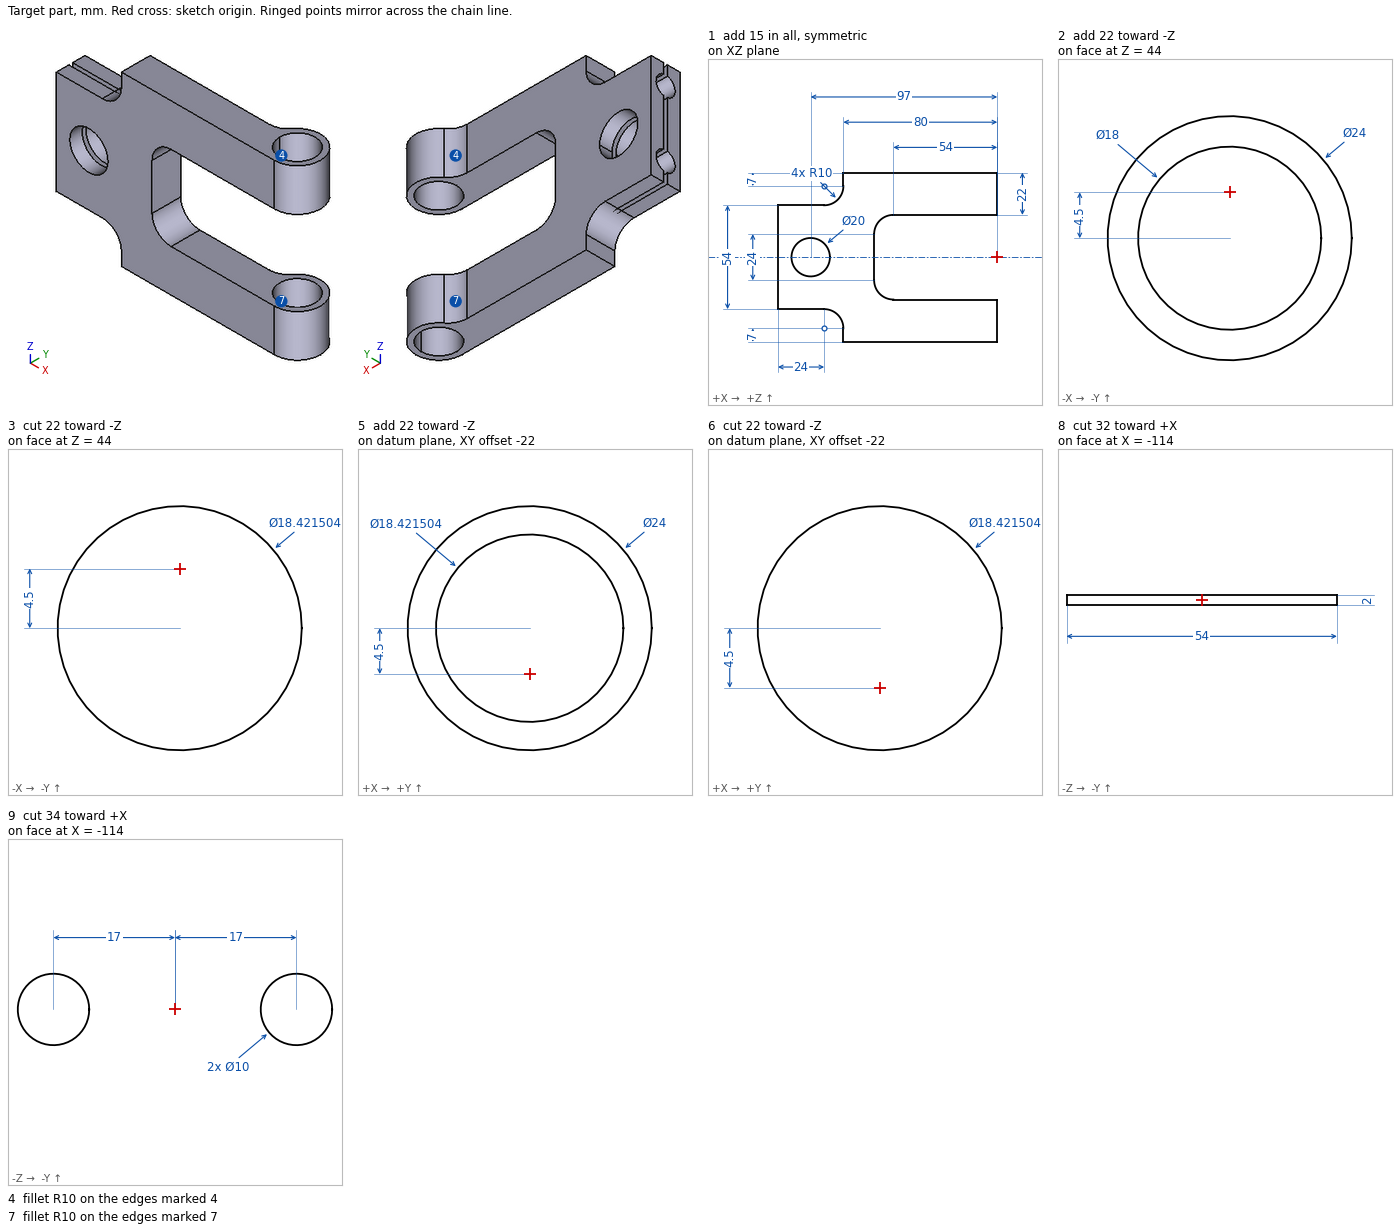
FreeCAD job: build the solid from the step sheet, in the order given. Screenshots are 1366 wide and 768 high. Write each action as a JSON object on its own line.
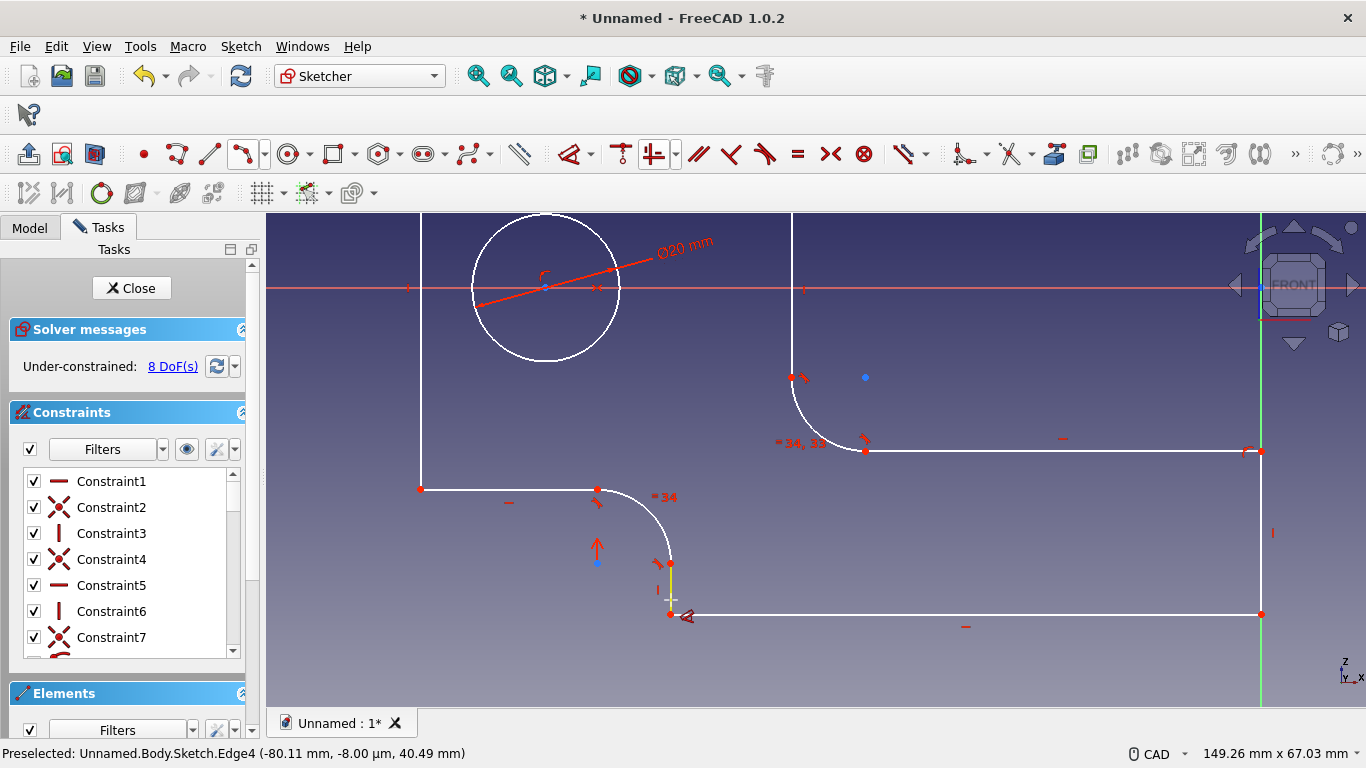
{"action": "left_click", "coordinate": [671, 599]}
{"action": "left_click", "coordinate": [637, 589]}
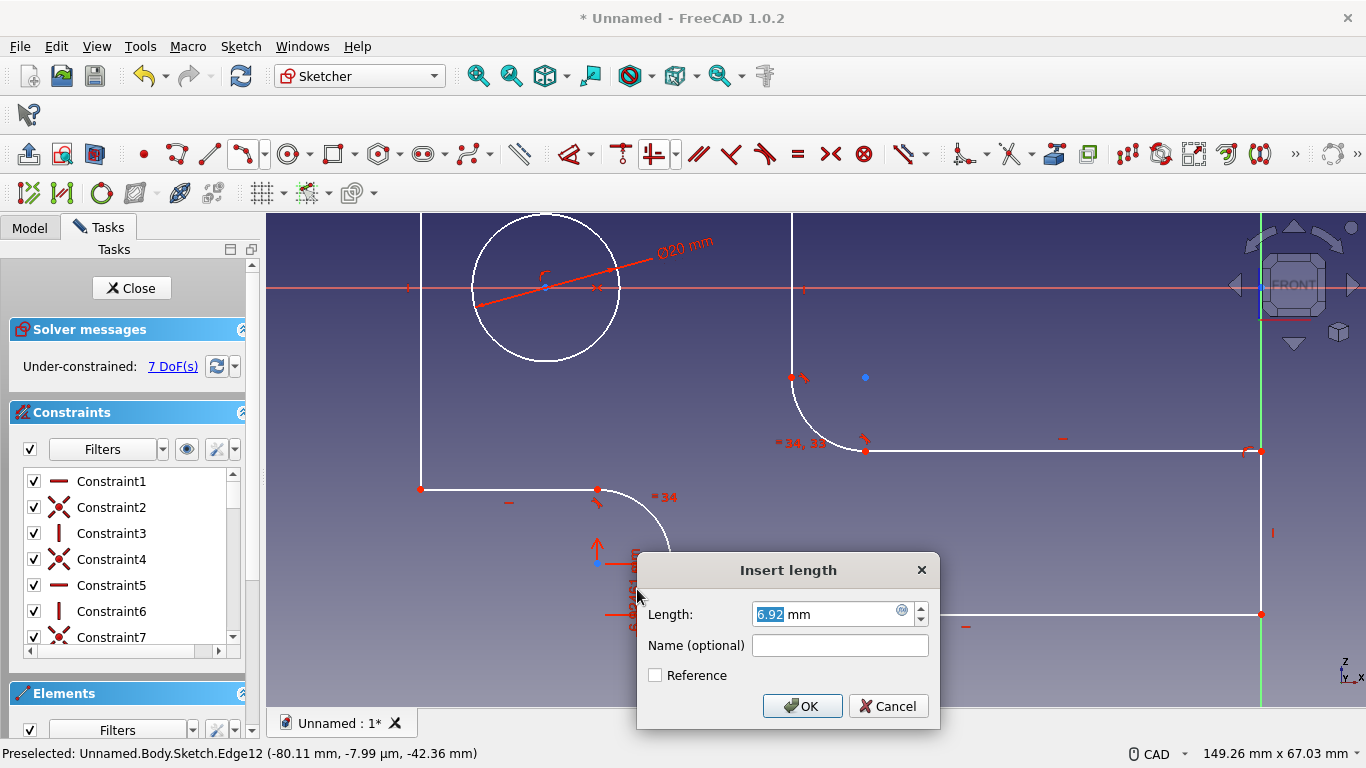
{"action": "type", "text": "7"}
{"action": "key", "text": "Return"}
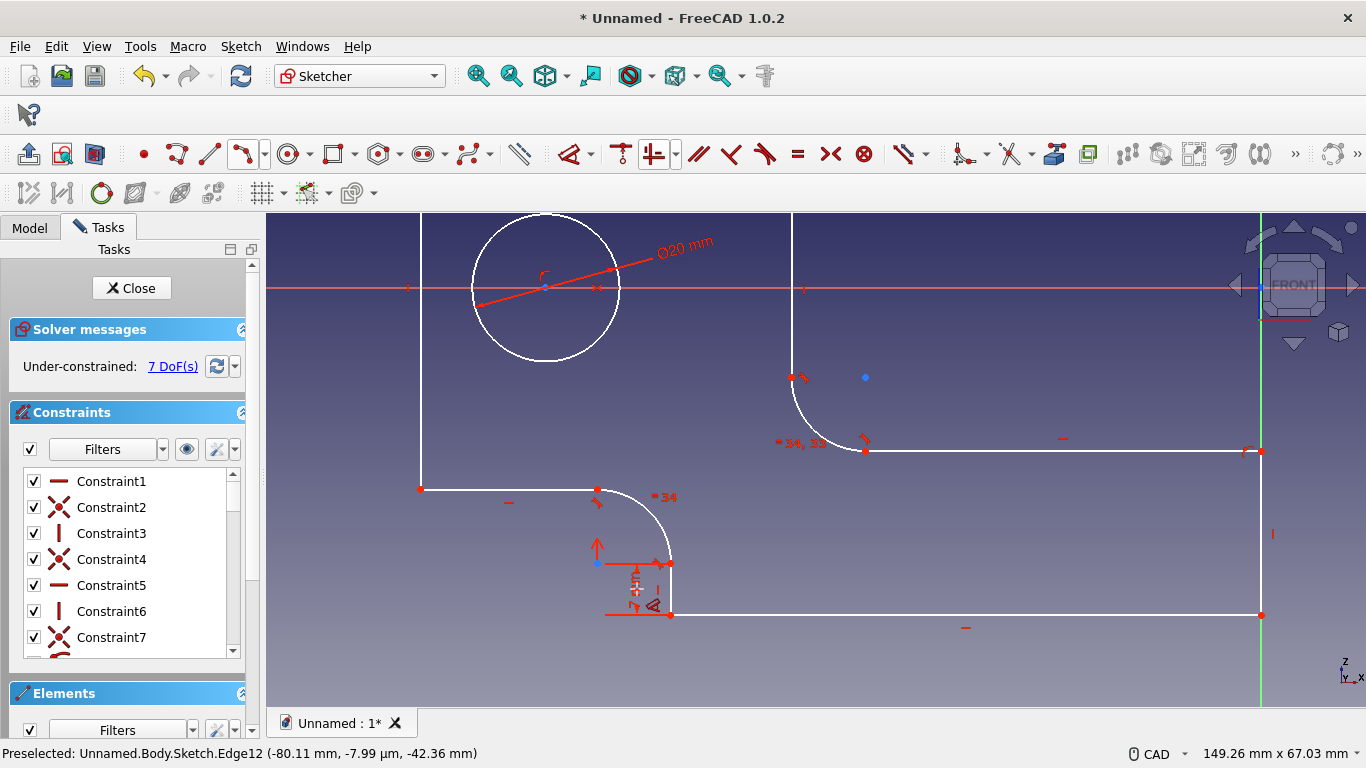
{"action": "left_click", "coordinate": [544, 490]}
{"action": "left_click", "coordinate": [509, 524]}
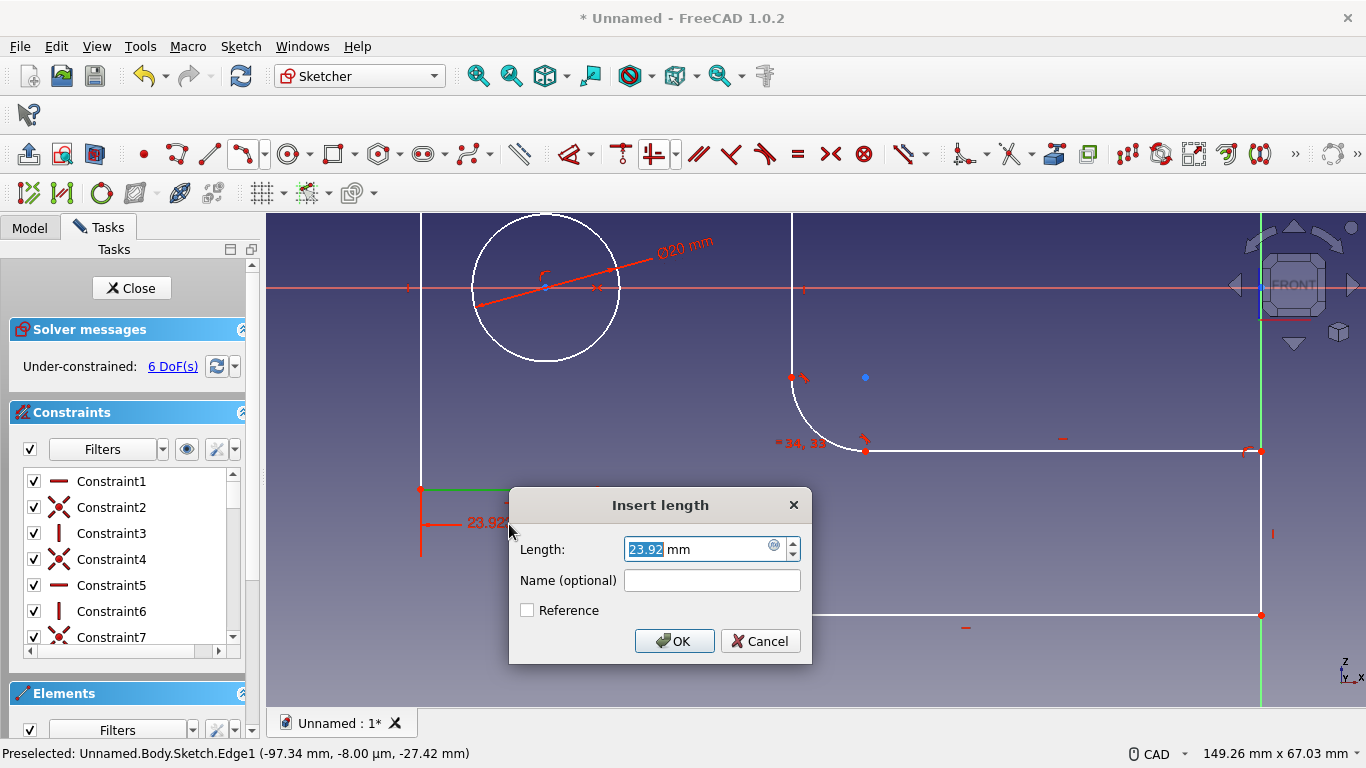
{"action": "type", "text": "24"}
{"action": "key", "text": "Return"}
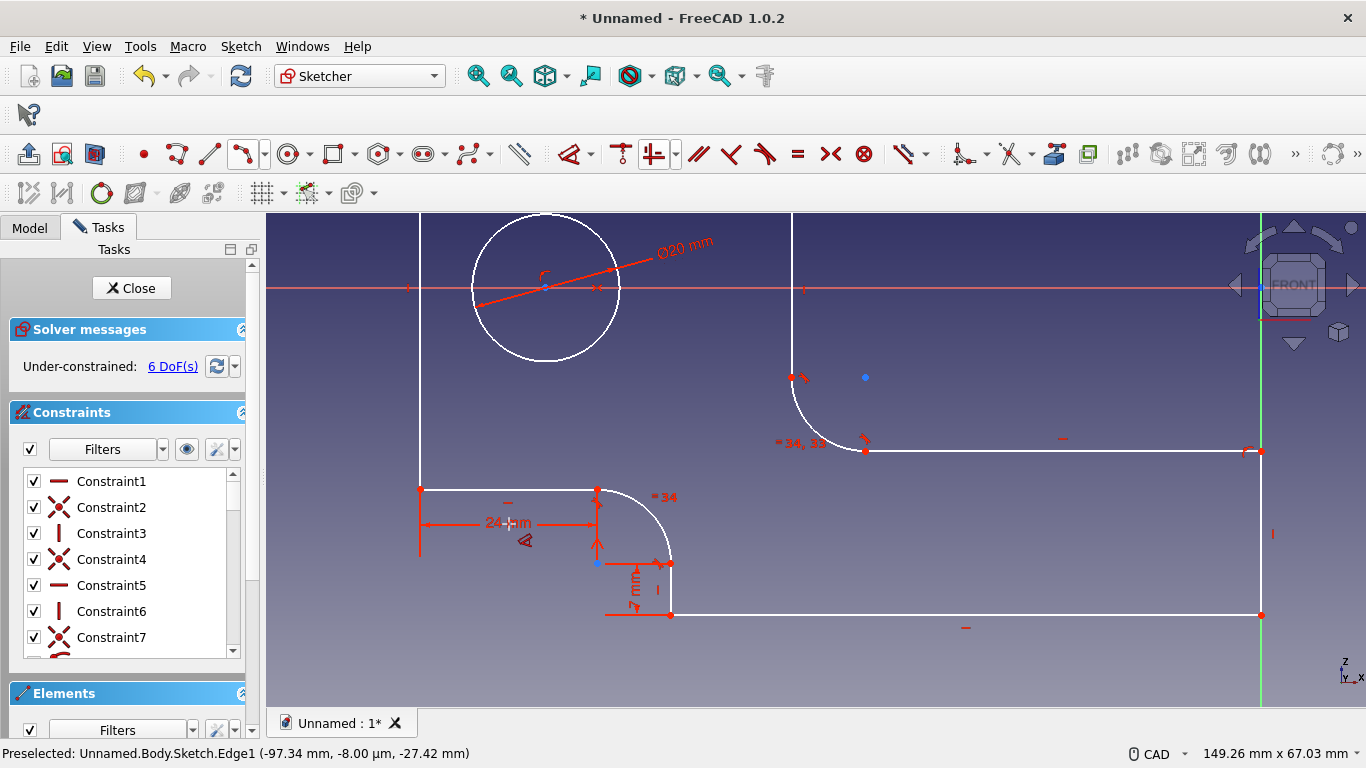
{"action": "left_click", "coordinate": [420, 369]}
{"action": "left_click", "coordinate": [386, 365]}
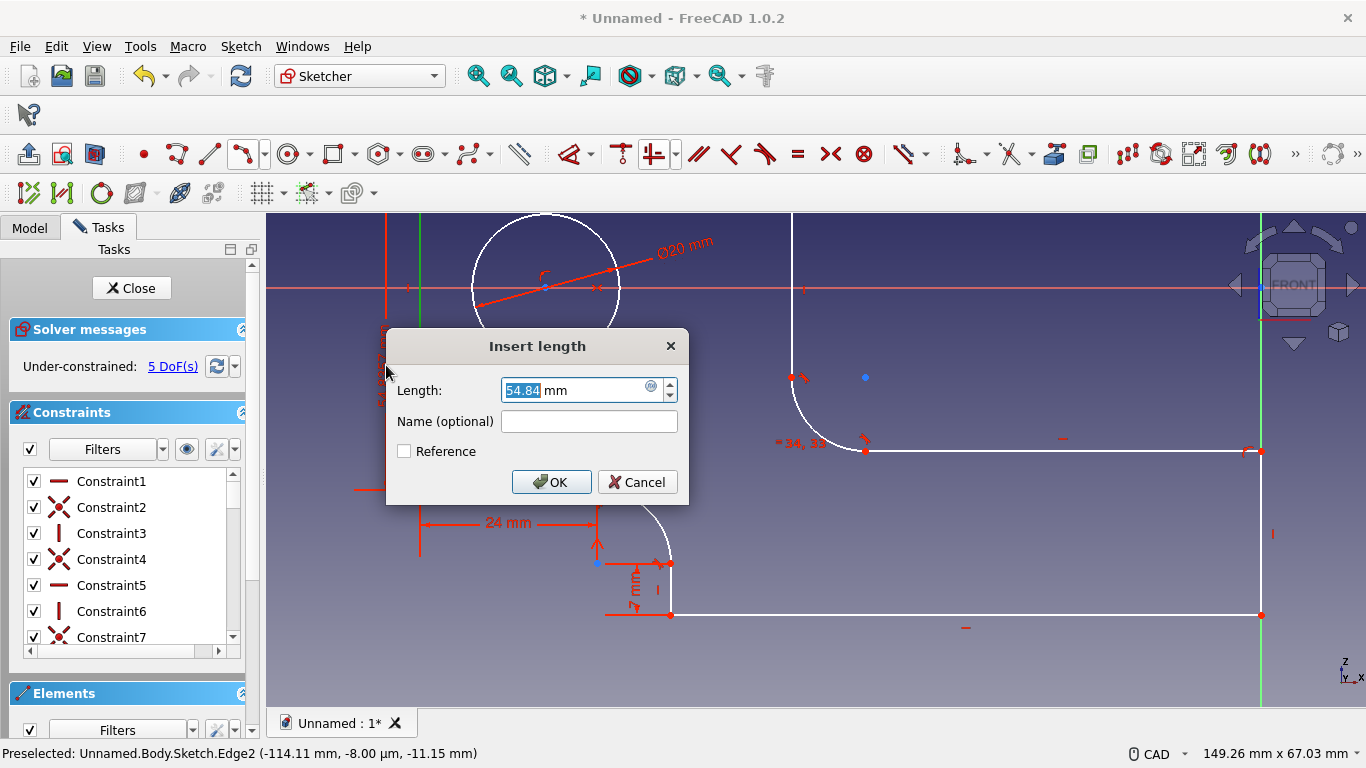
{"action": "type", "text": "54"}
{"action": "key", "text": "Return"}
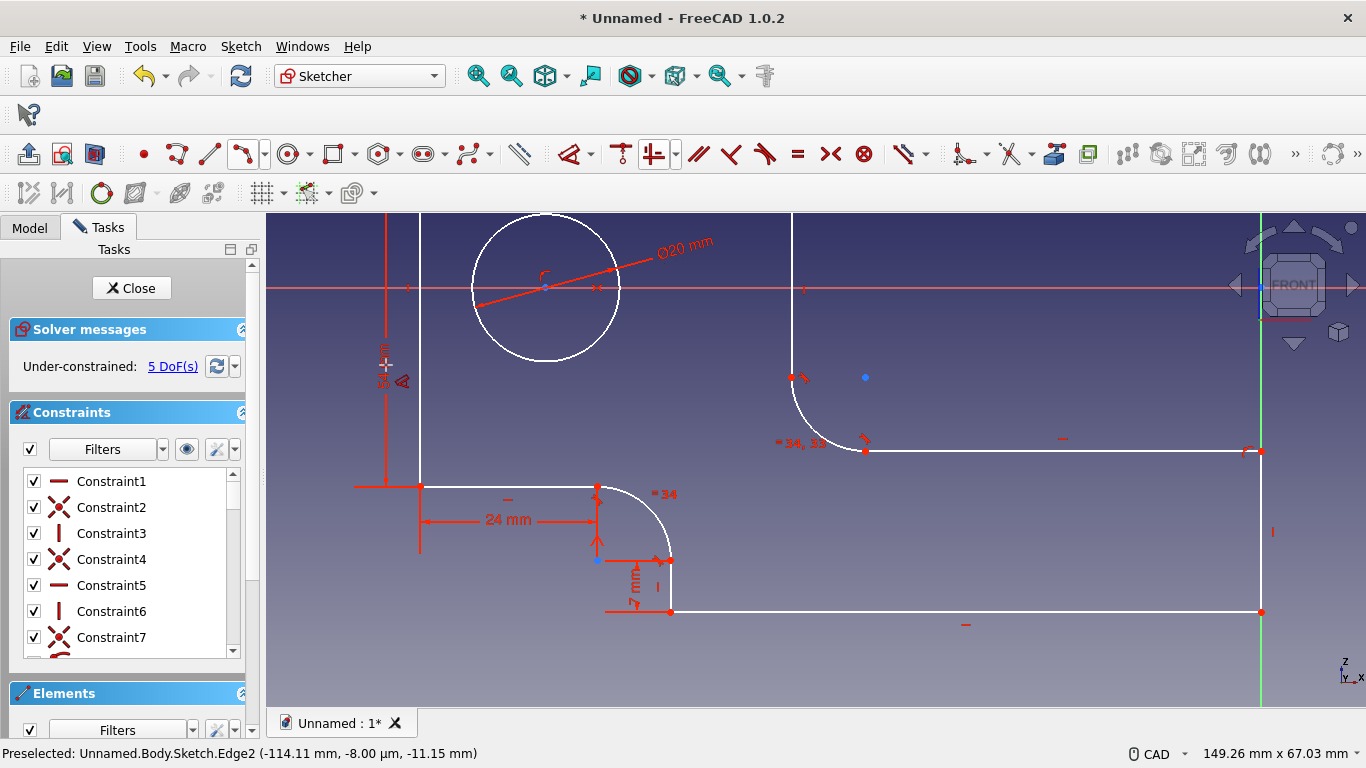
{"action": "scroll", "coordinate": [671, 600], "scroll_direction": "down", "scroll_amount": 4}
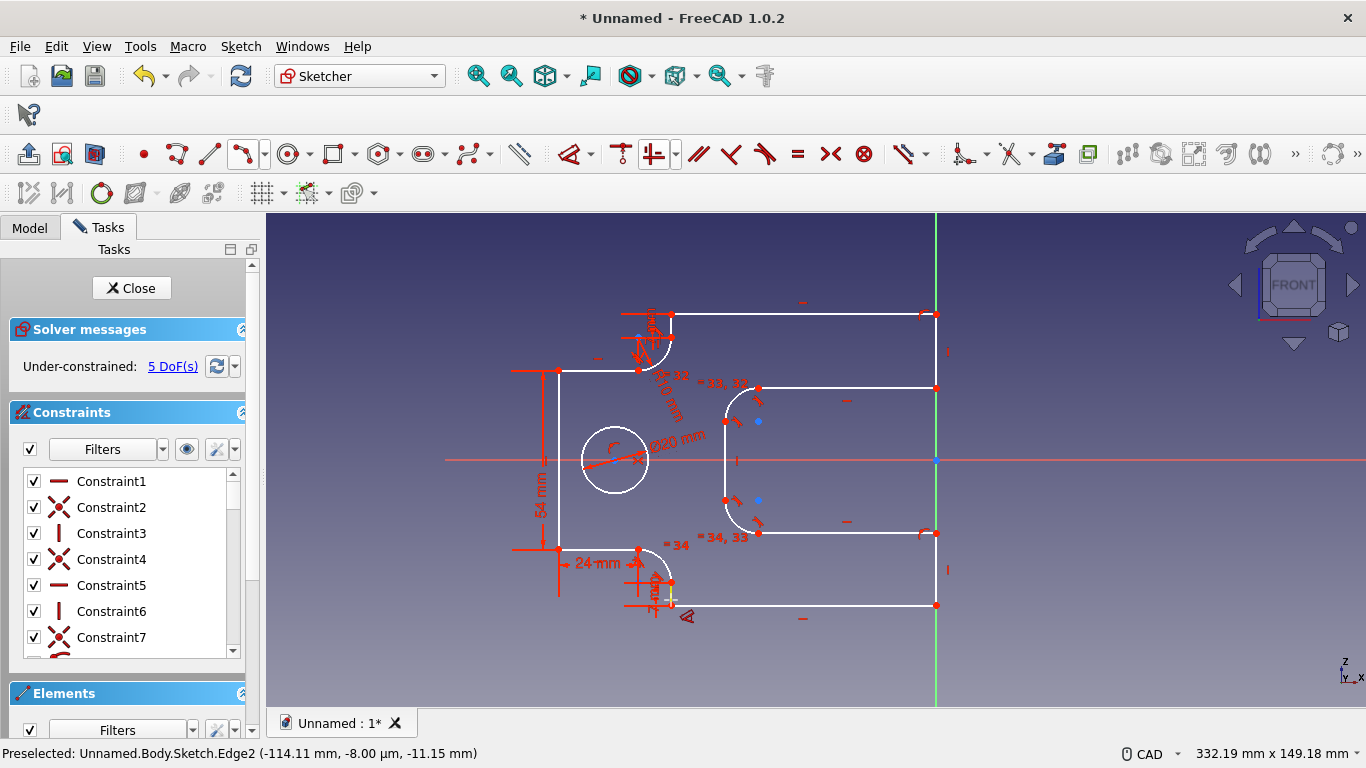
{"action": "left_click", "coordinate": [751, 314]}
{"action": "left_click", "coordinate": [804, 280]}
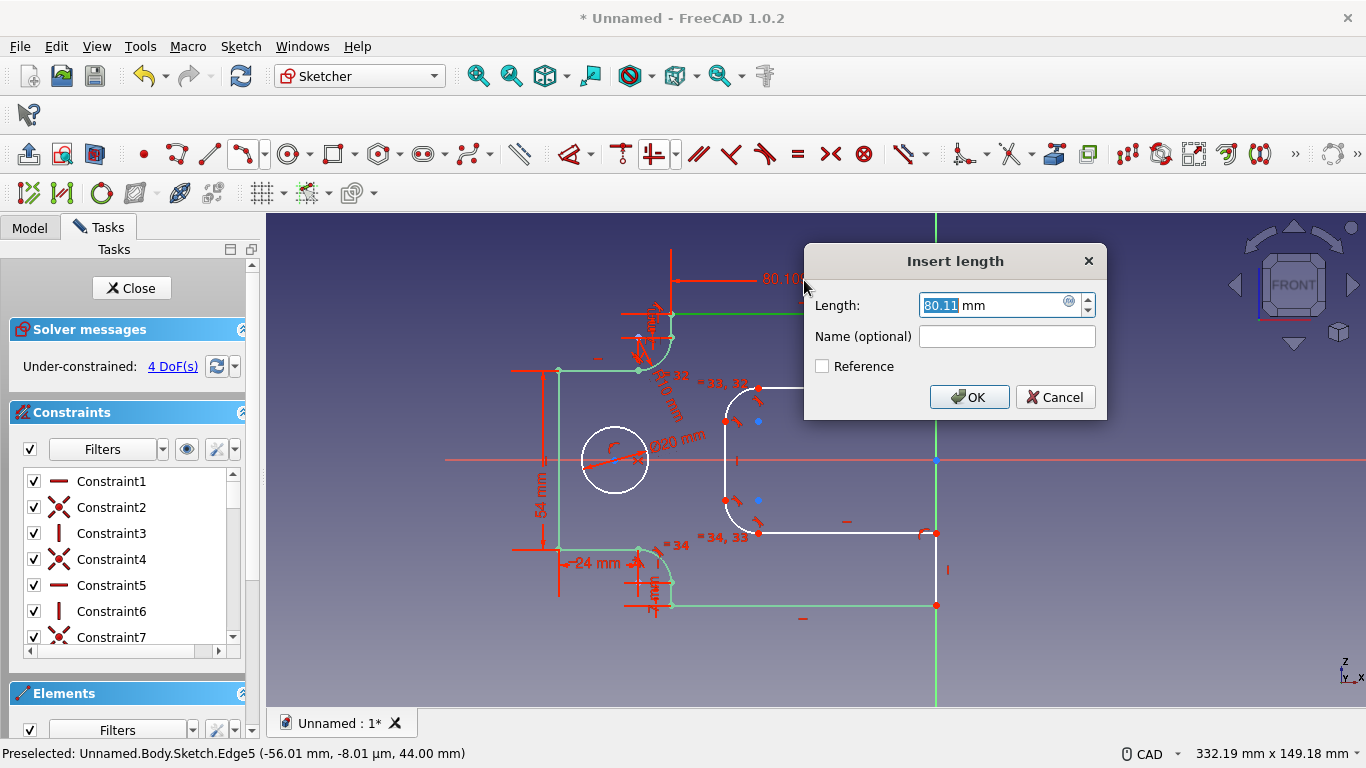
{"action": "type", "text": "80"}
{"action": "key", "text": "Return"}